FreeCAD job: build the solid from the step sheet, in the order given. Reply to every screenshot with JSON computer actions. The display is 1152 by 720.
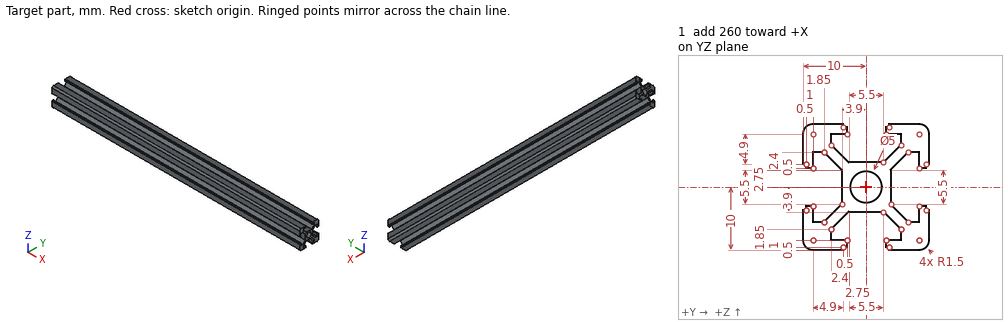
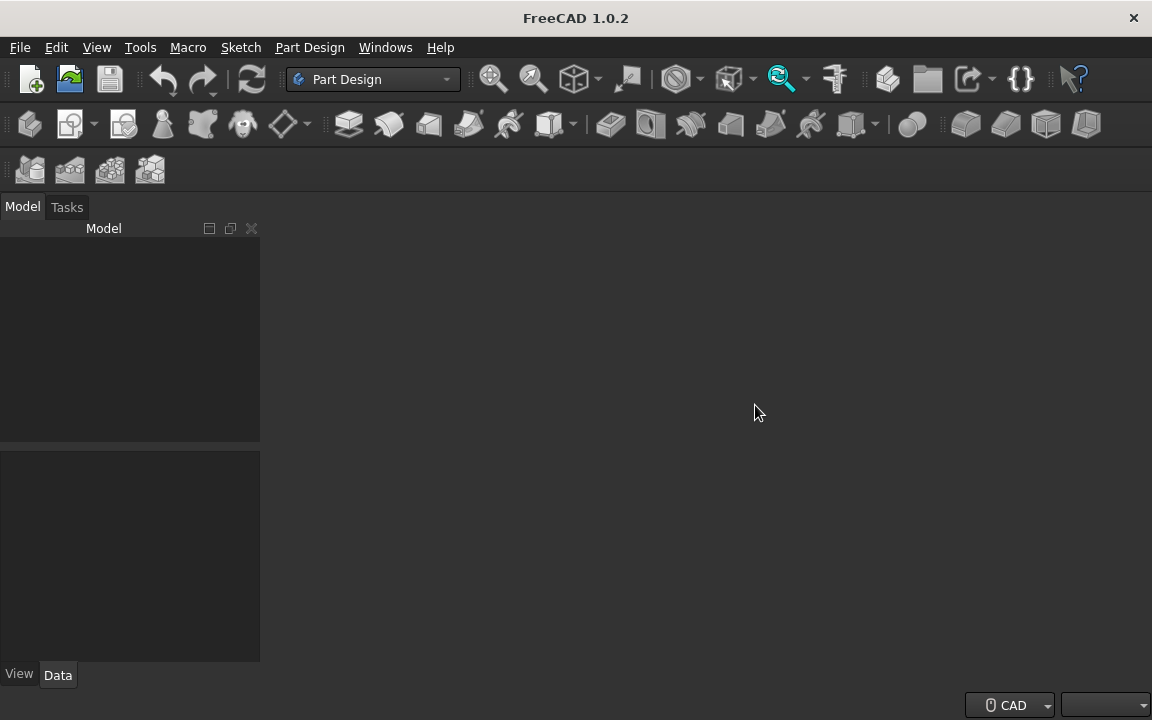
{"action": "key", "text": "ctrl+n"}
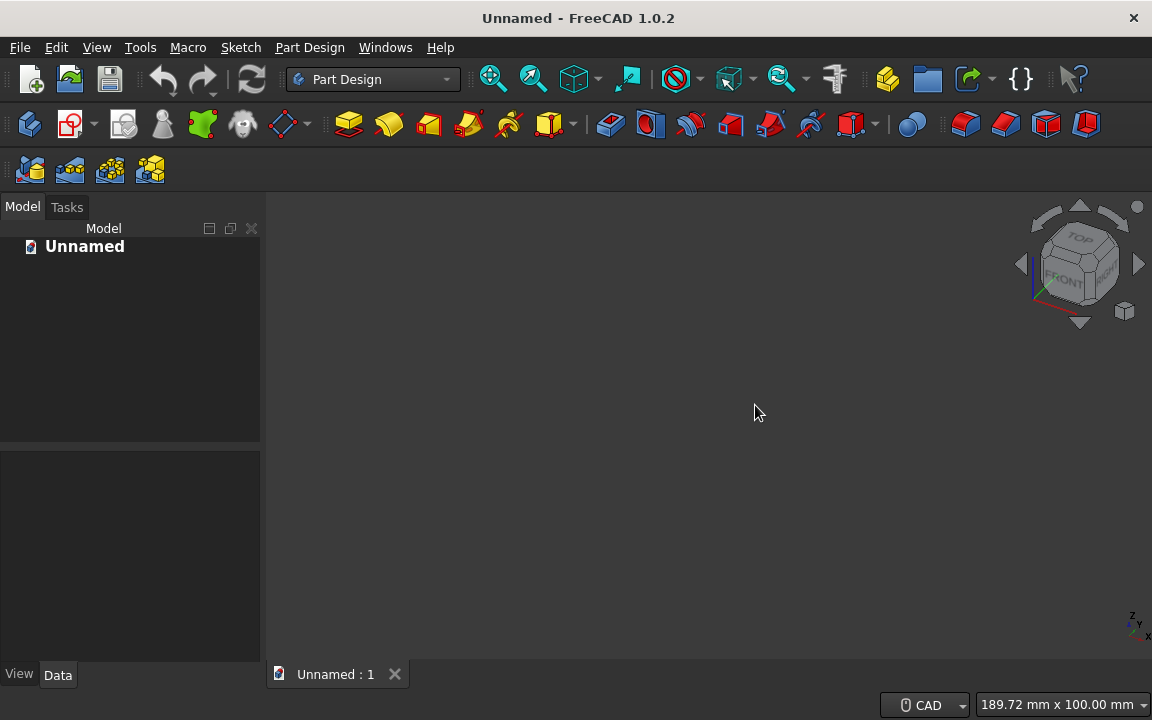
{"action": "left_click", "coordinate": [70, 124]}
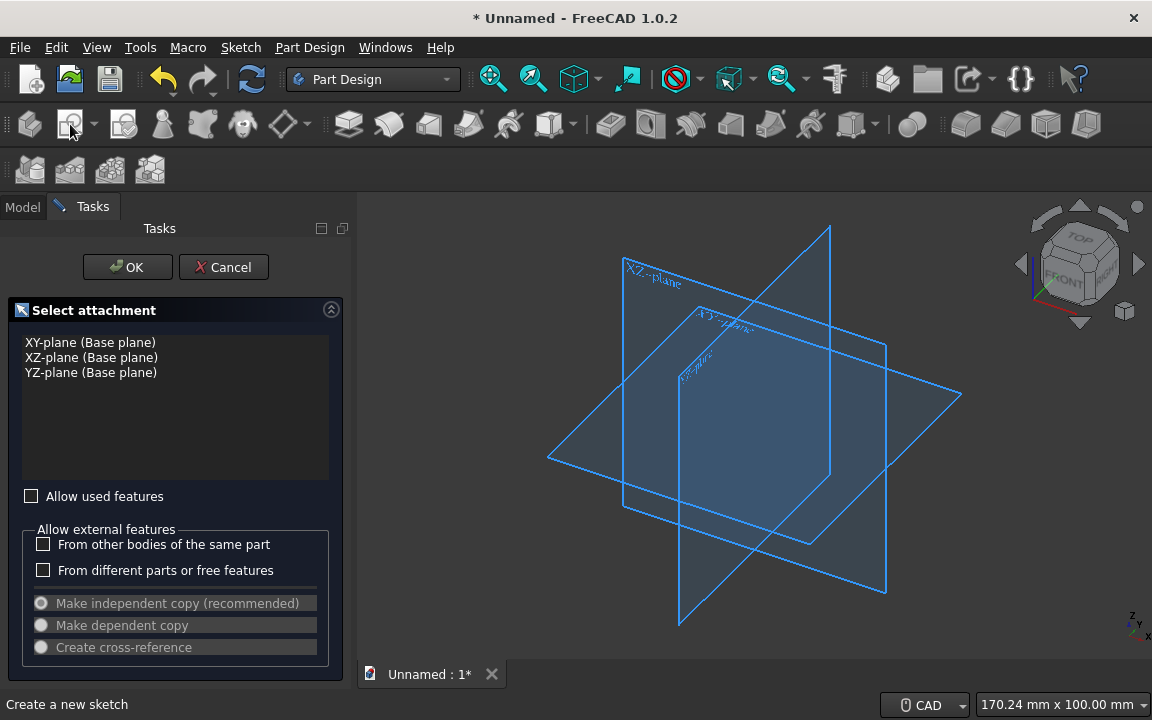
{"action": "left_click", "coordinate": [82, 372]}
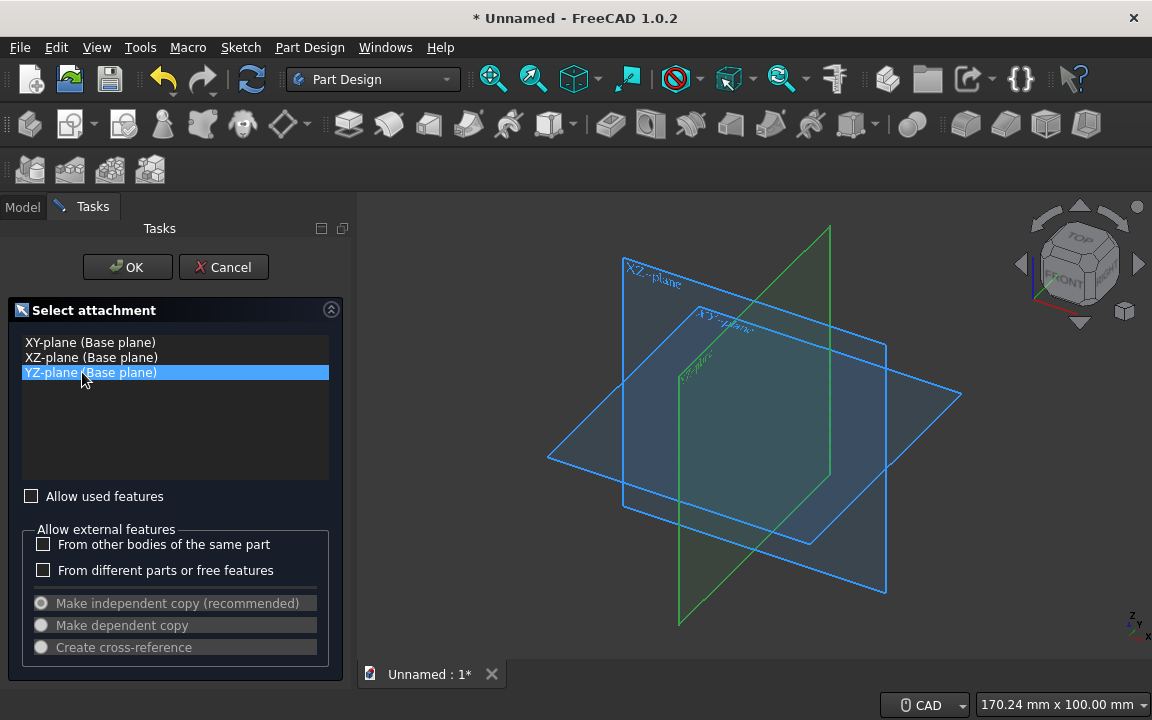
{"action": "left_click", "coordinate": [128, 267]}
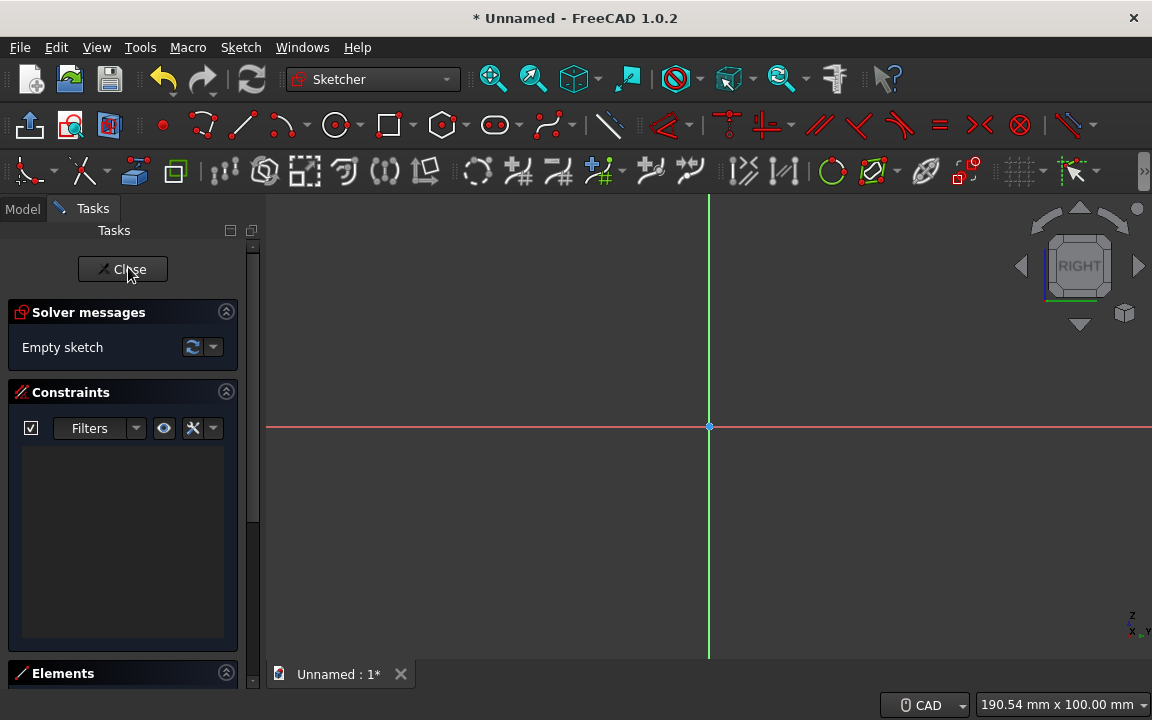
{"action": "scroll", "coordinate": [739, 427], "scroll_direction": "up", "scroll_amount": 6}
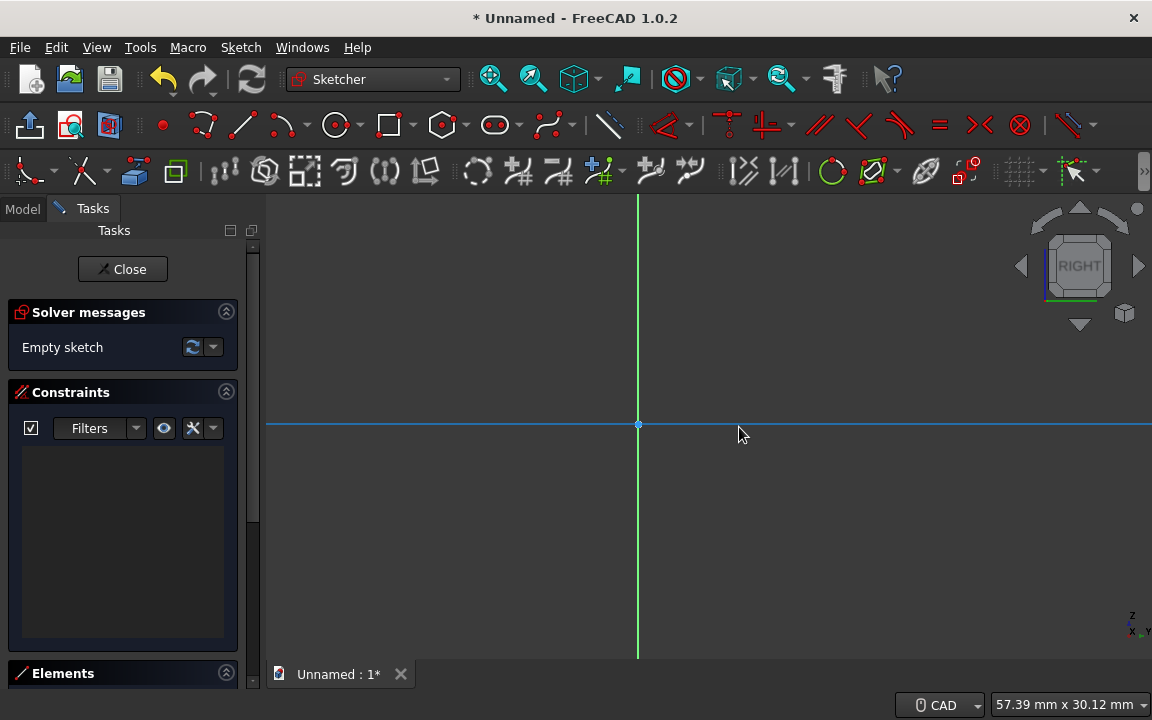
{"action": "left_click", "coordinate": [204, 126]}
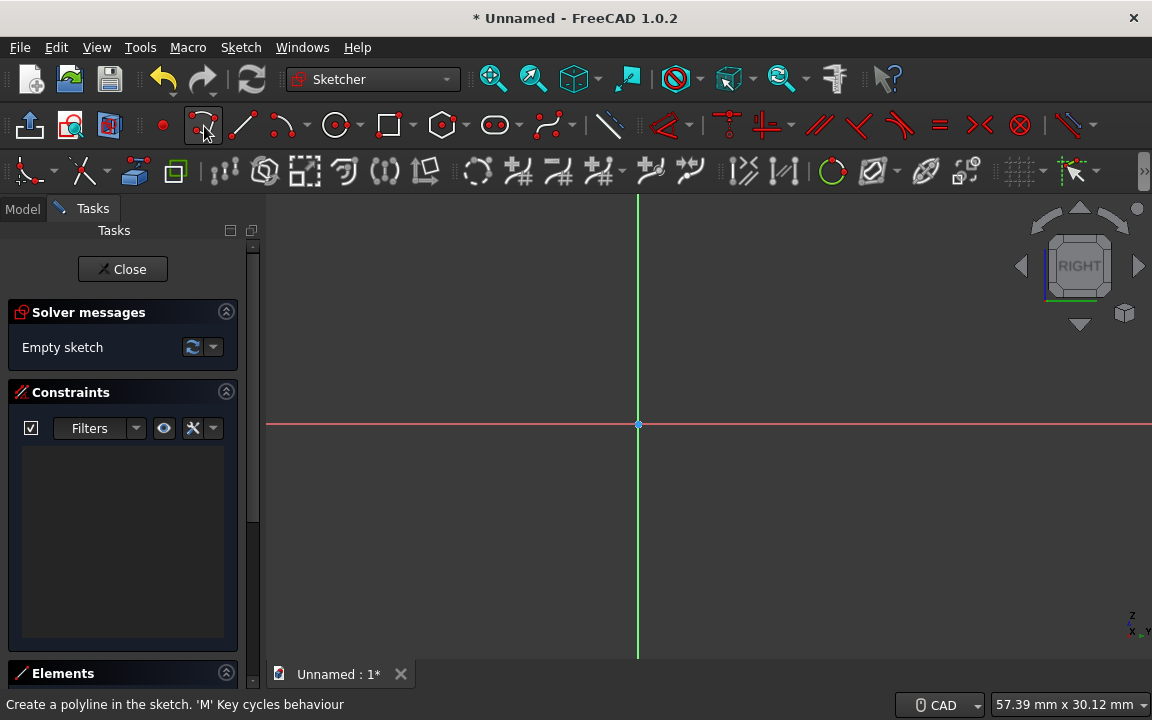
{"action": "left_click", "coordinate": [484, 293]}
{"action": "left_click", "coordinate": [484, 369]}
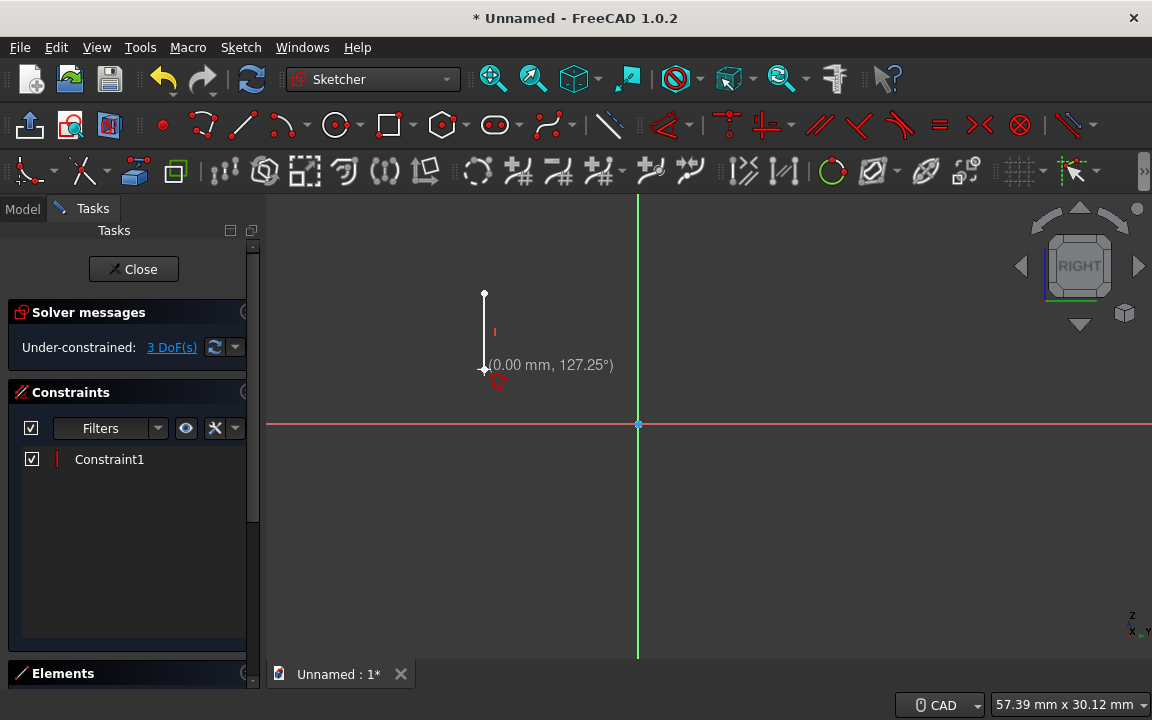
{"action": "scroll", "coordinate": [491, 369], "scroll_direction": "up", "scroll_amount": 4}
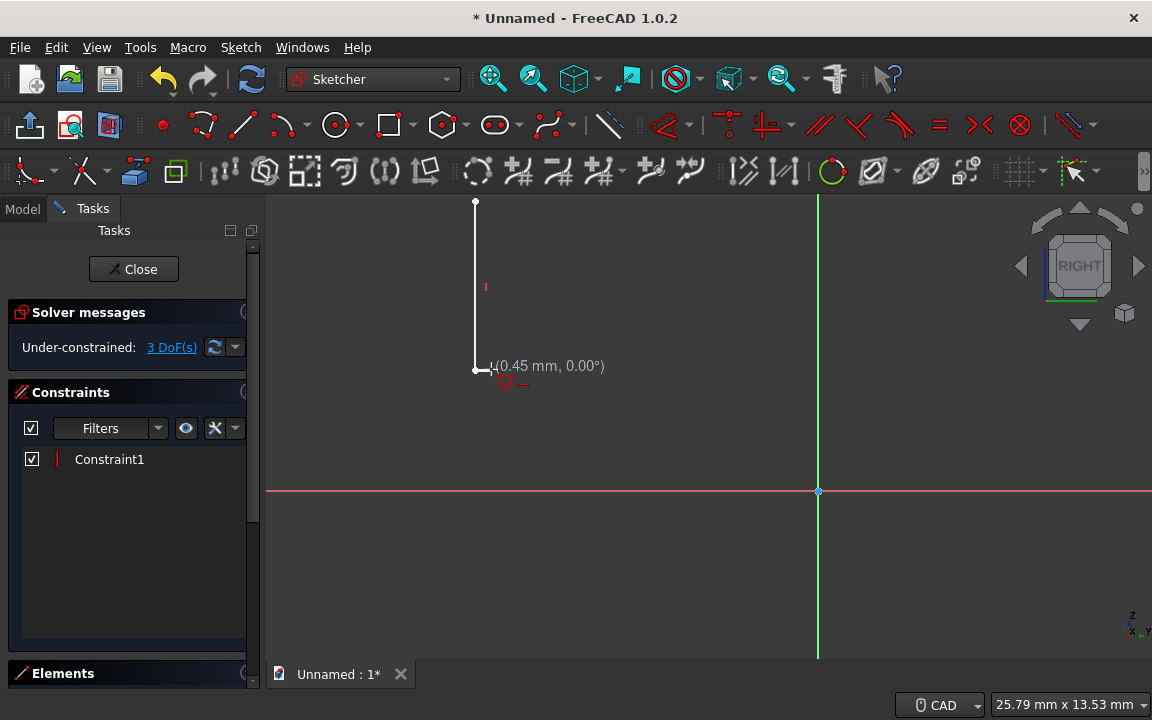
{"action": "left_click", "coordinate": [492, 369]}
{"action": "left_click", "coordinate": [492, 385]}
{"action": "left_click", "coordinate": [526, 385]}
{"action": "left_click", "coordinate": [526, 302]}
{"action": "left_click", "coordinate": [590, 302]}
{"action": "left_click", "coordinate": [684, 397]}
{"action": "left_click", "coordinate": [684, 586]}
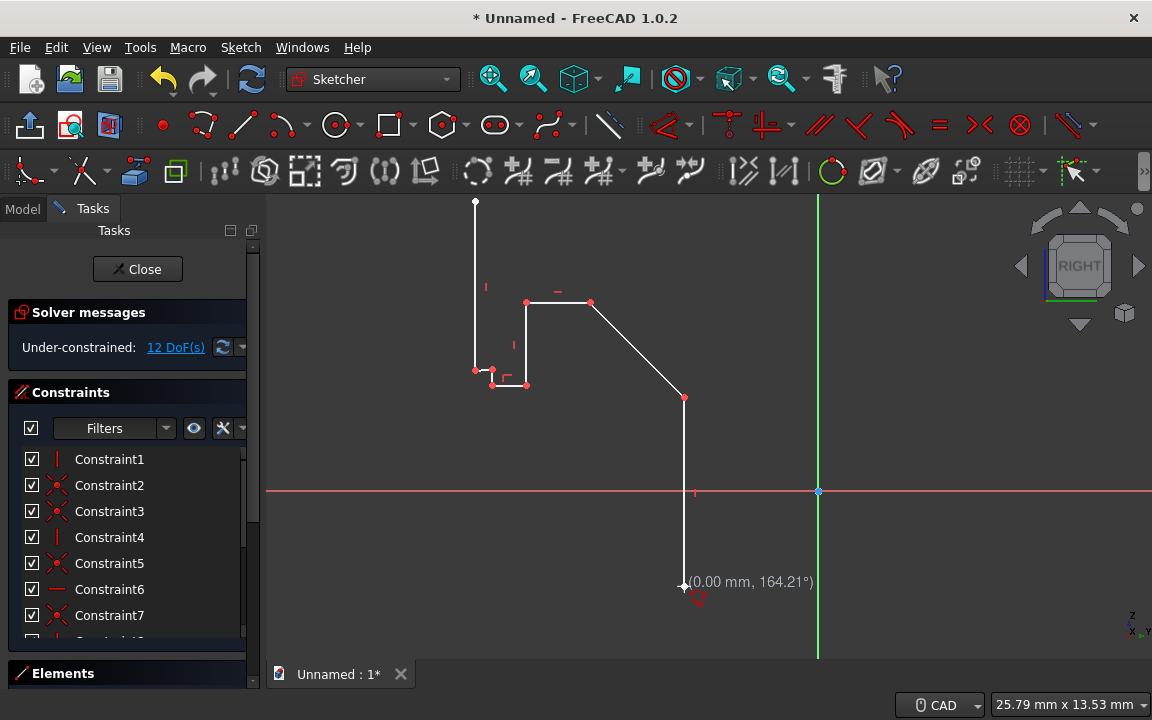
{"action": "scroll", "coordinate": [496, 374], "scroll_direction": "down", "scroll_amount": 4}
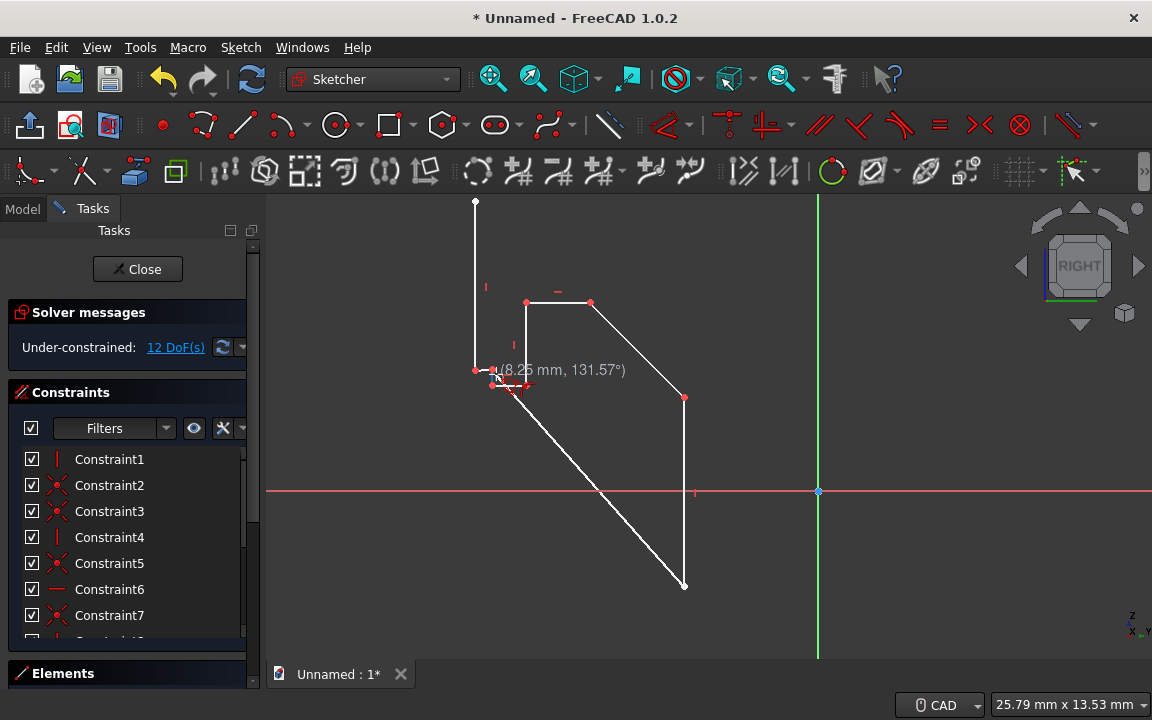
{"action": "left_click", "coordinate": [538, 512]}
{"action": "left_click", "coordinate": [510, 512]}
{"action": "left_click", "coordinate": [510, 475]}
{"action": "left_click", "coordinate": [494, 475]}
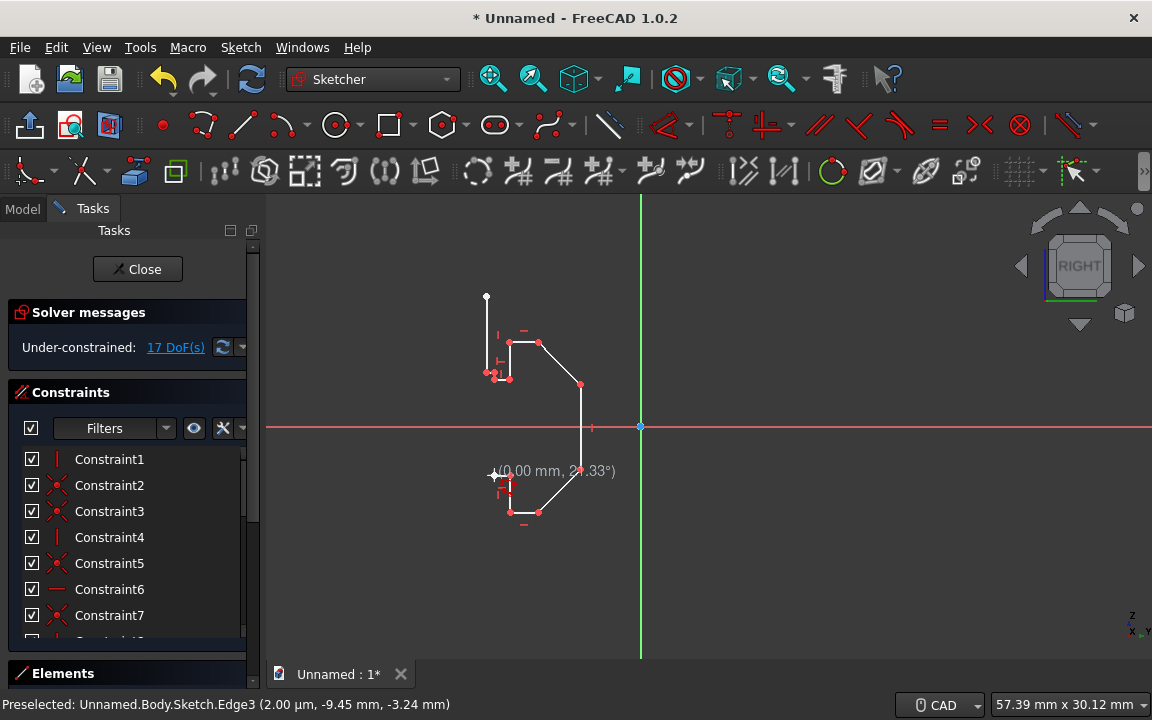
{"action": "scroll", "coordinate": [494, 483], "scroll_direction": "up", "scroll_amount": 4}